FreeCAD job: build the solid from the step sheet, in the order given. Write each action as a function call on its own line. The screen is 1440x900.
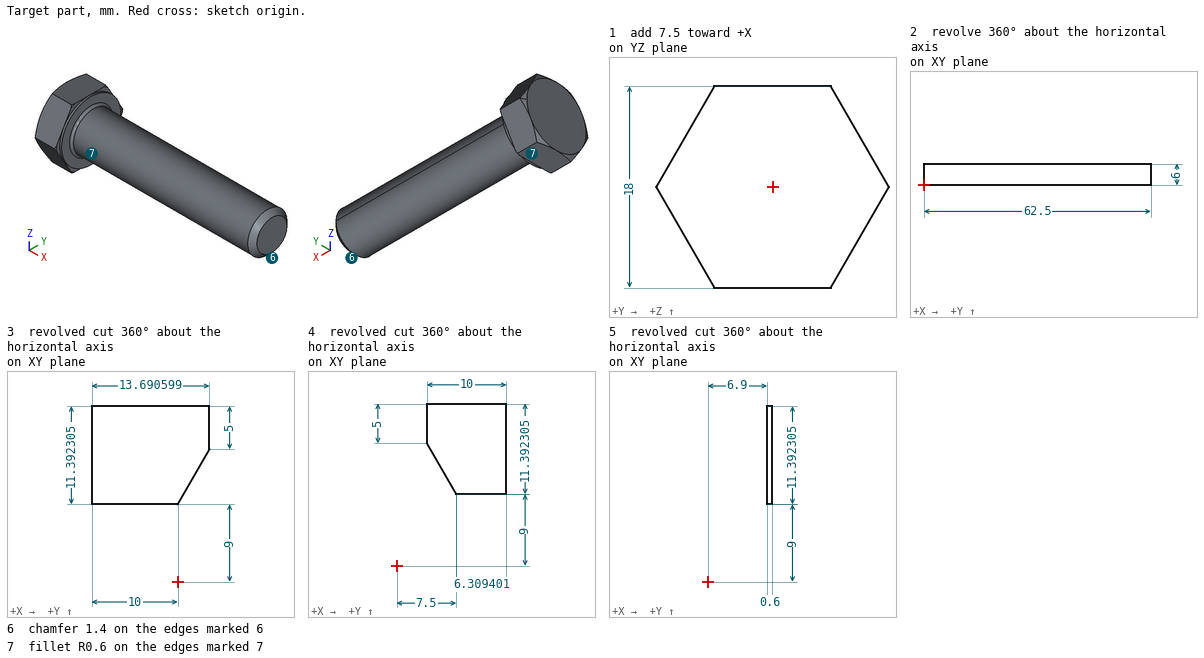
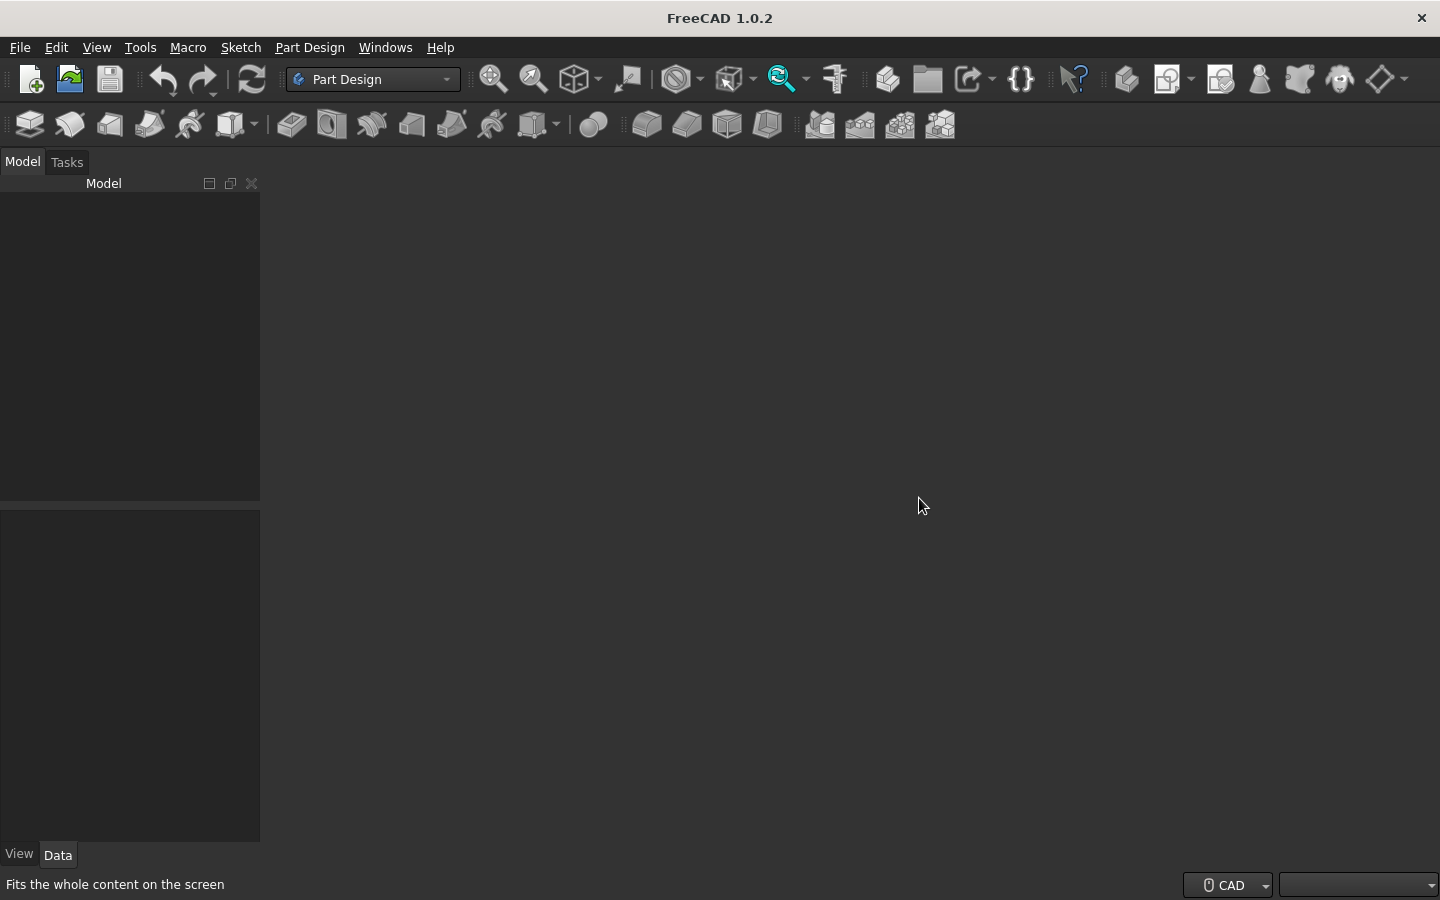
click(30, 80)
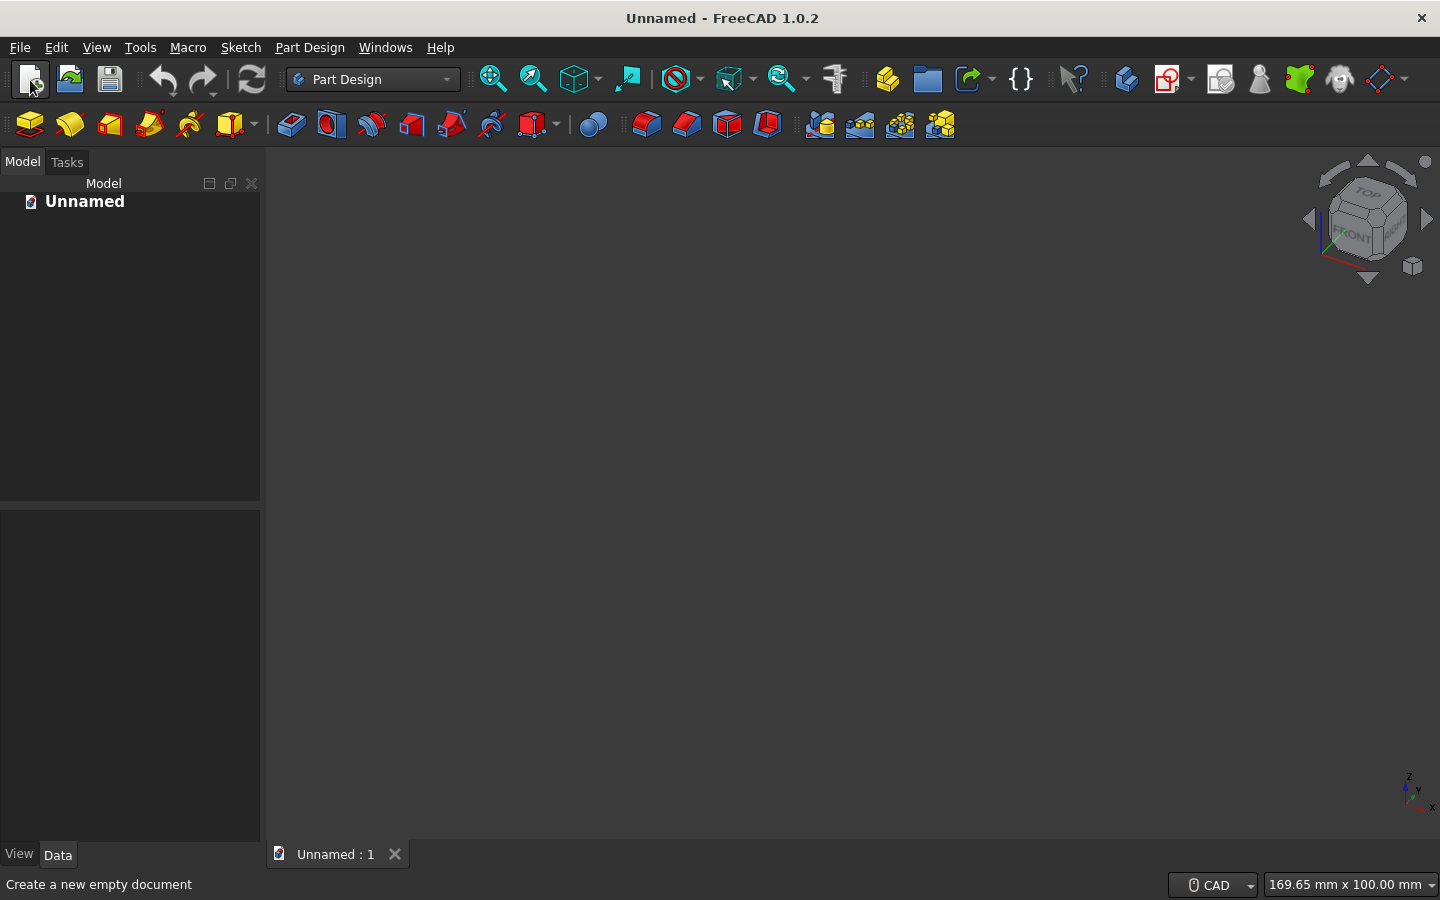
click(1168, 80)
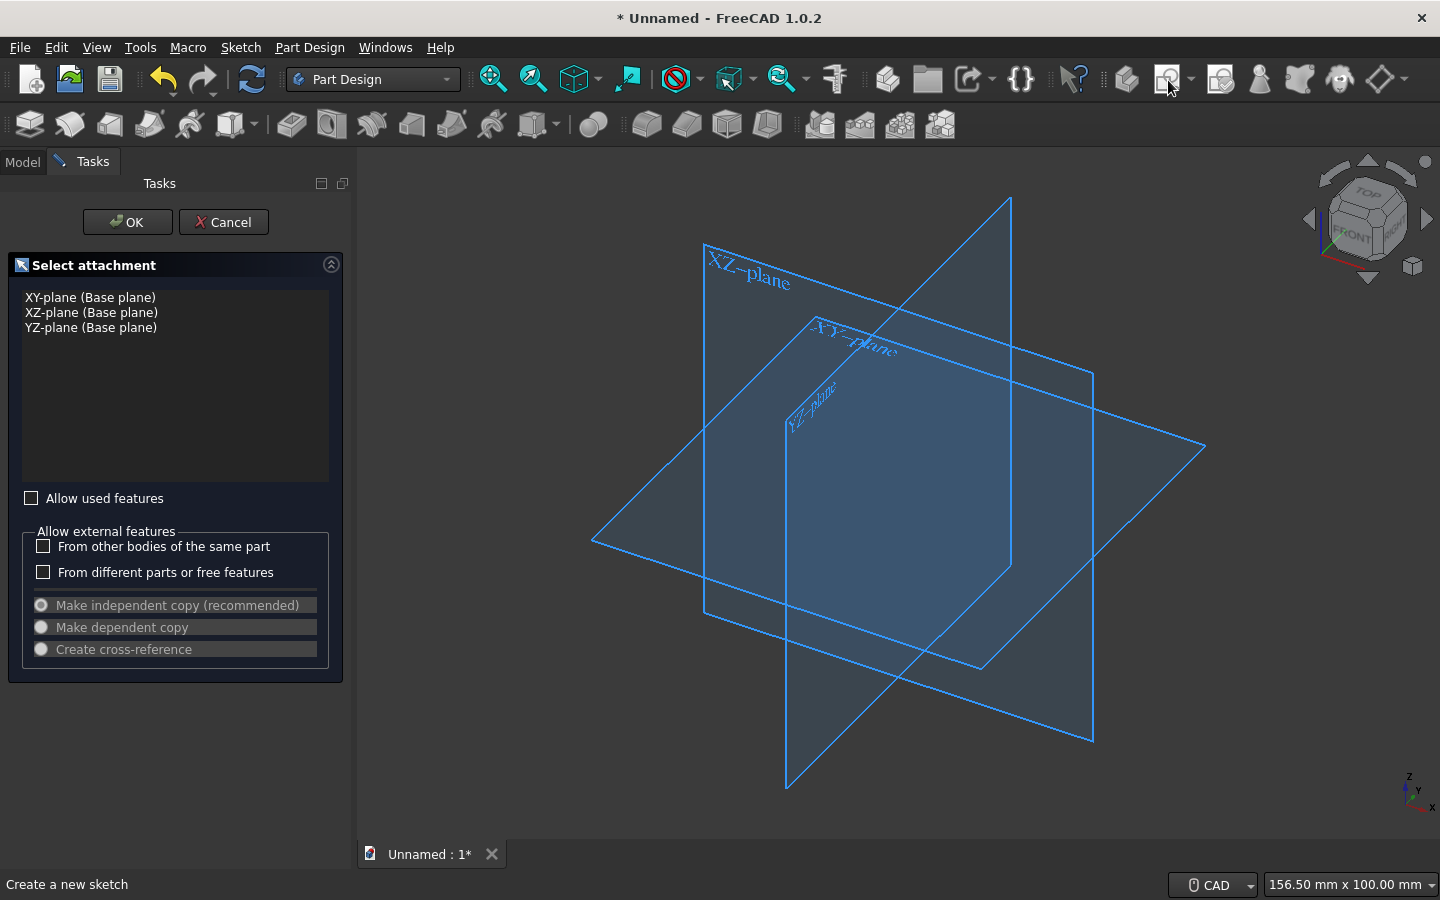
click(82, 328)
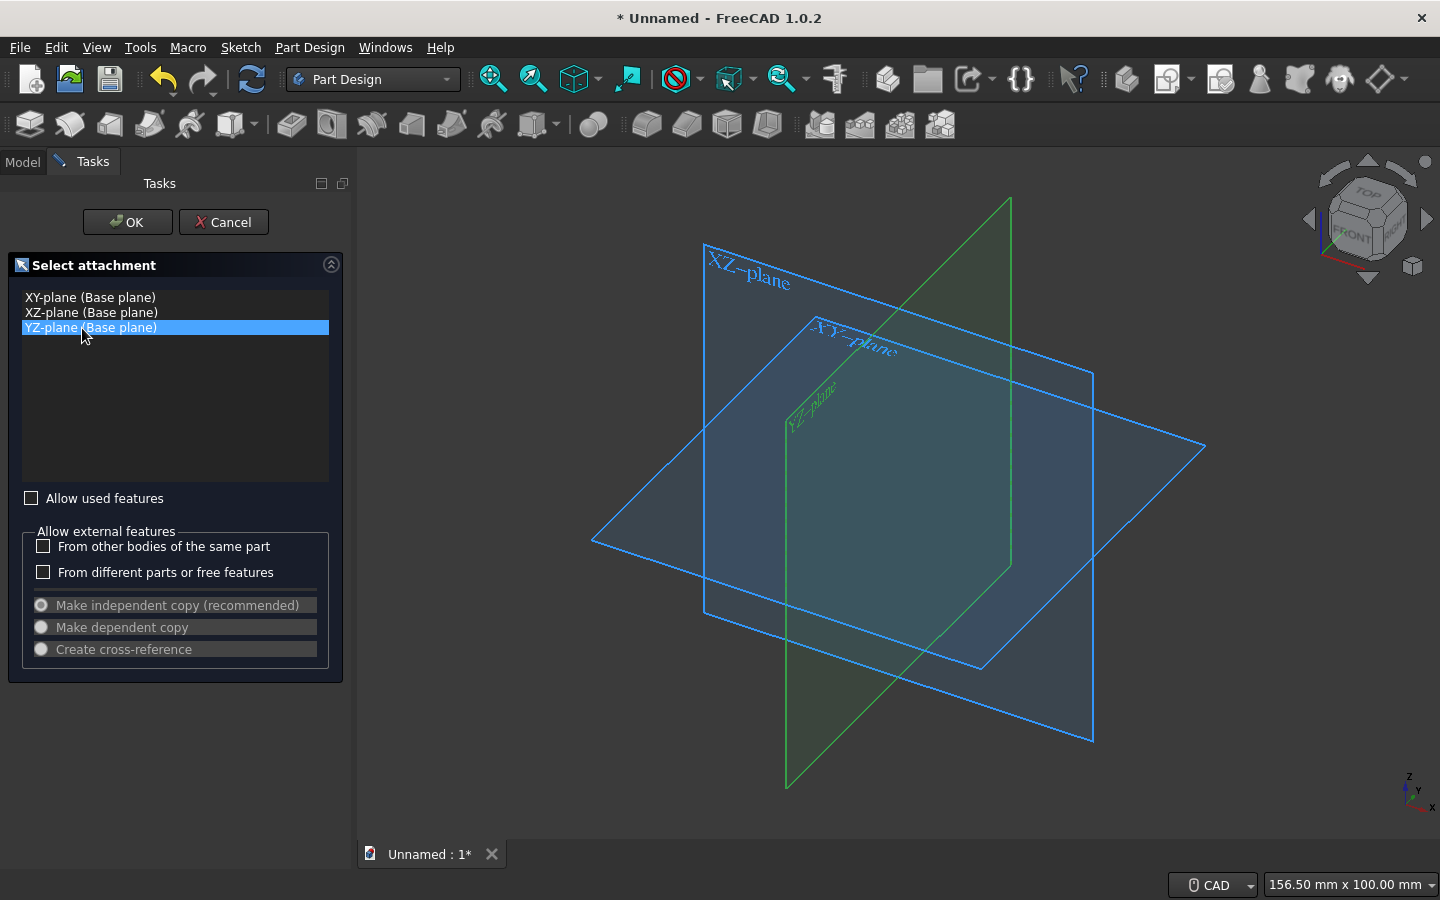
click(128, 222)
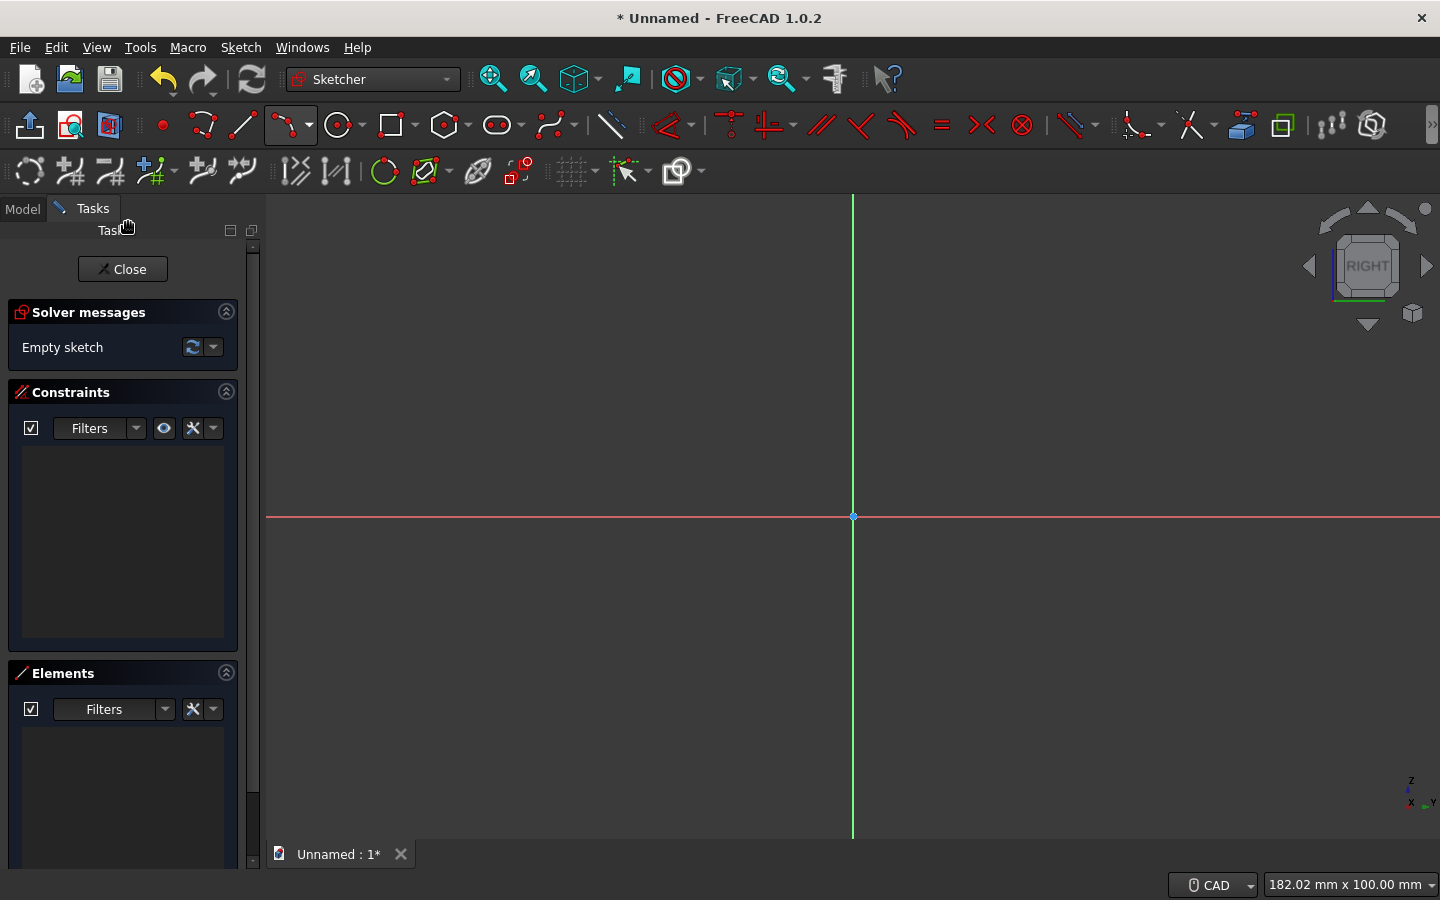
scroll(883, 516, up, 6)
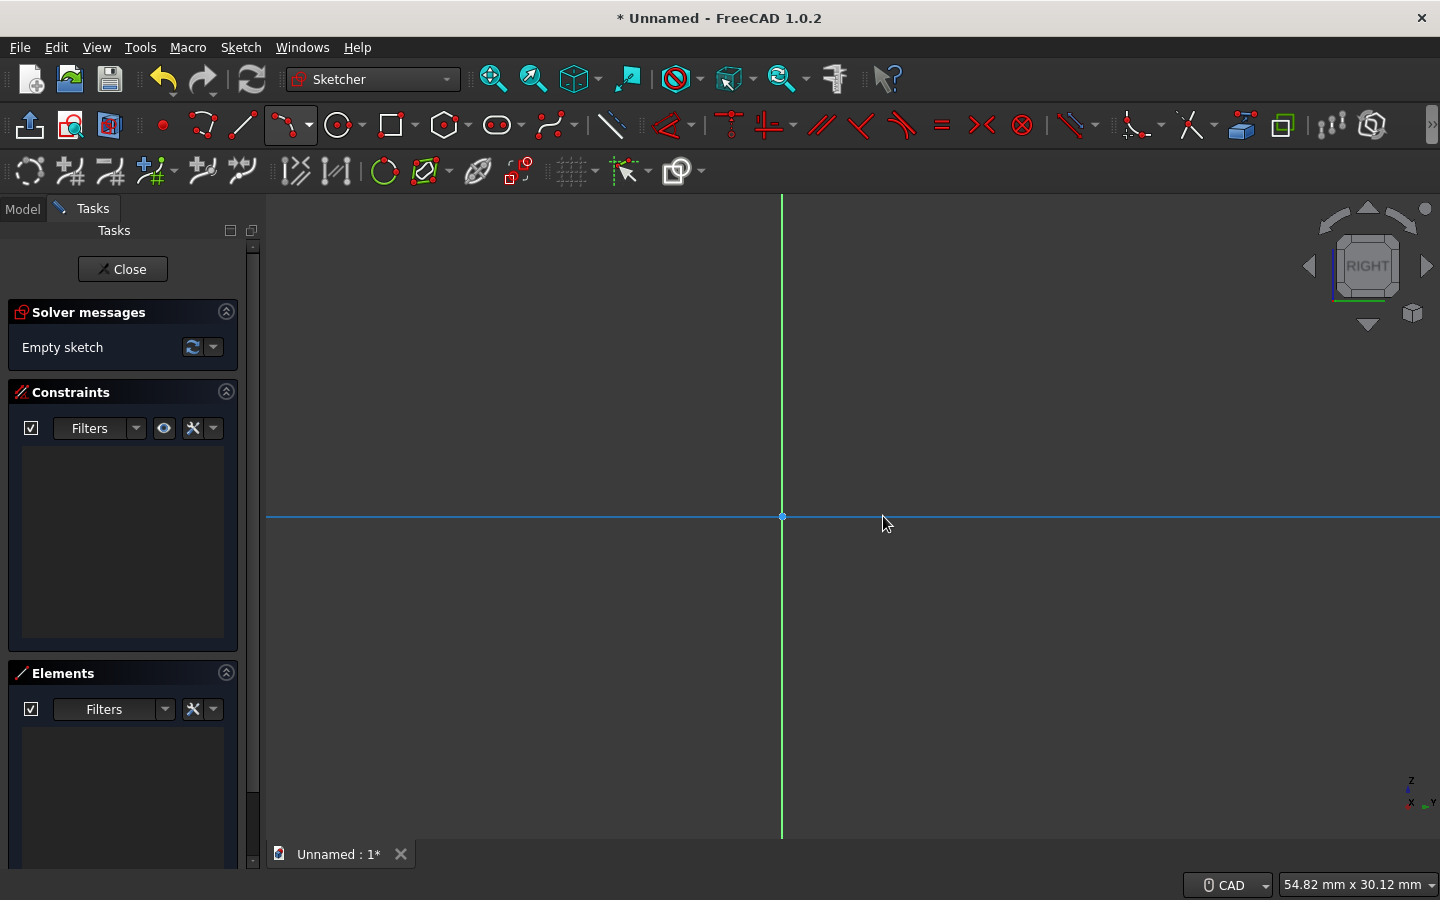
click(444, 126)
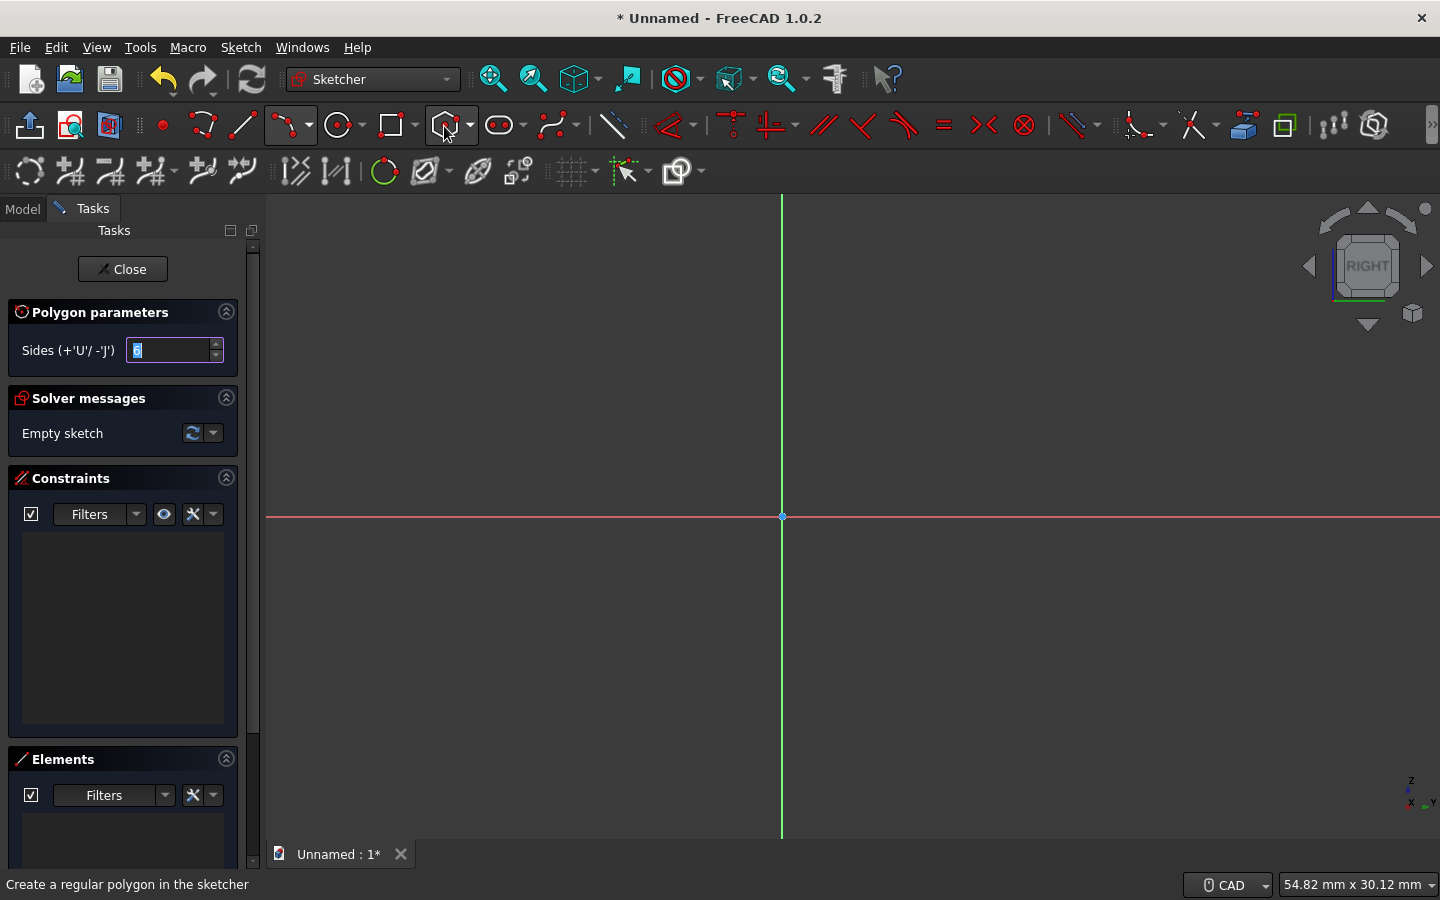
click(782, 516)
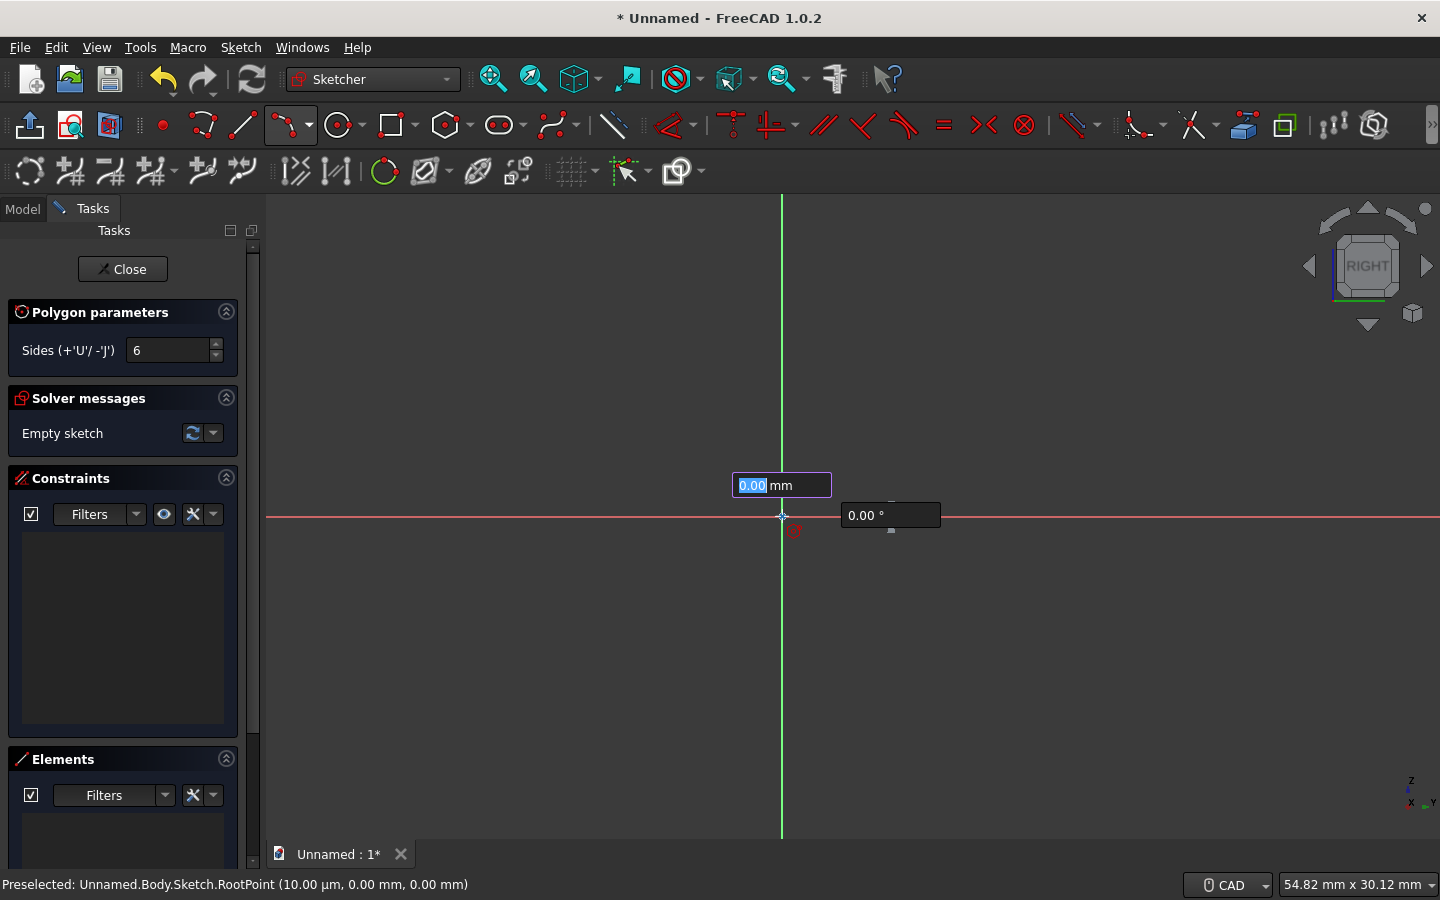
click(1005, 516)
key(Escape)